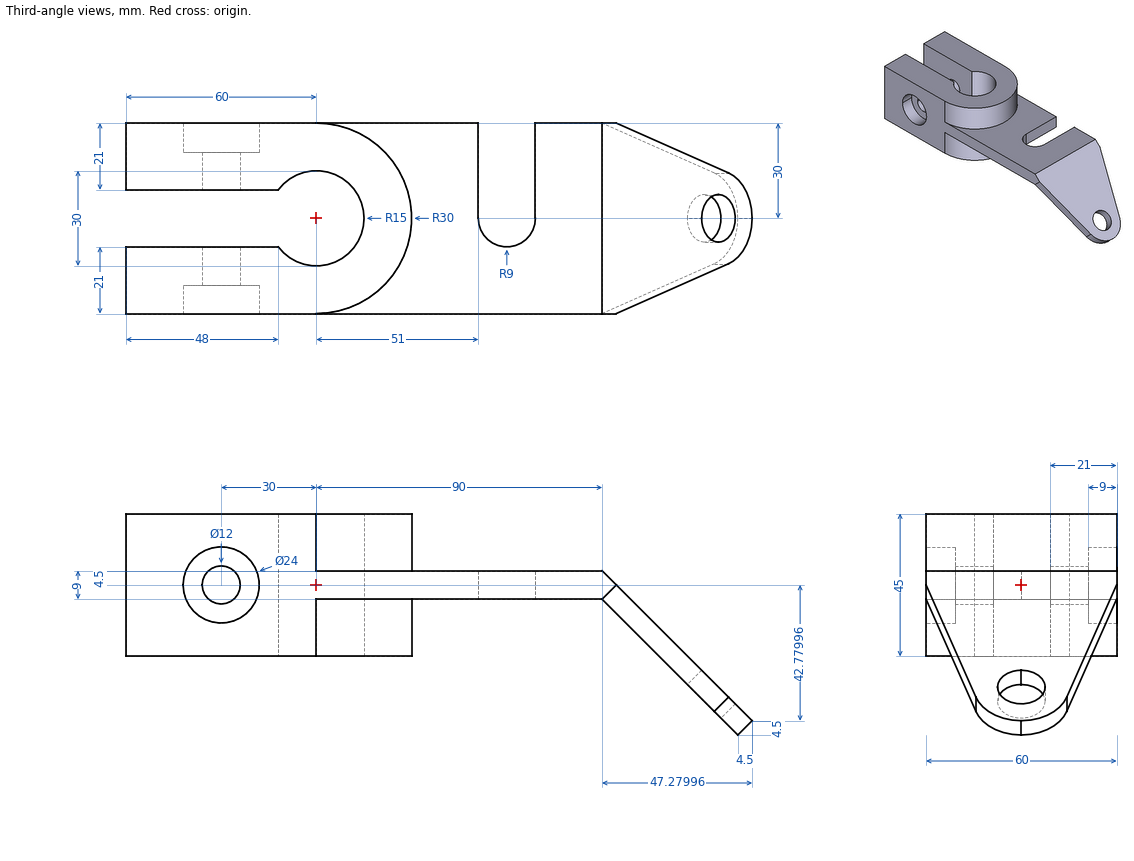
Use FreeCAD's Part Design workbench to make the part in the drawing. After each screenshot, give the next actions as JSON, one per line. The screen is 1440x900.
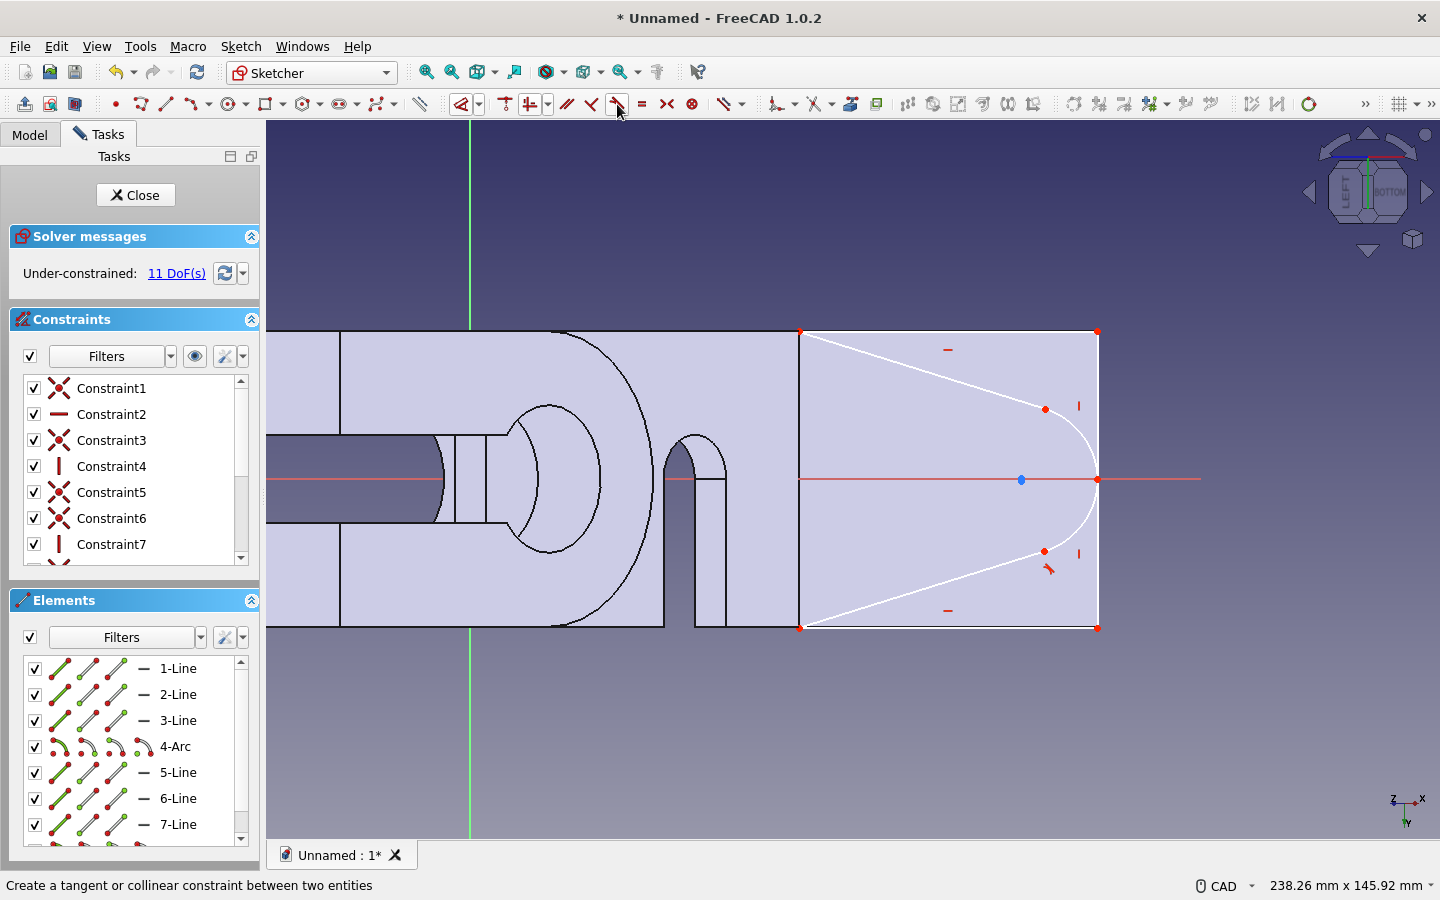
{"action": "left_click", "coordinate": [1098, 583]}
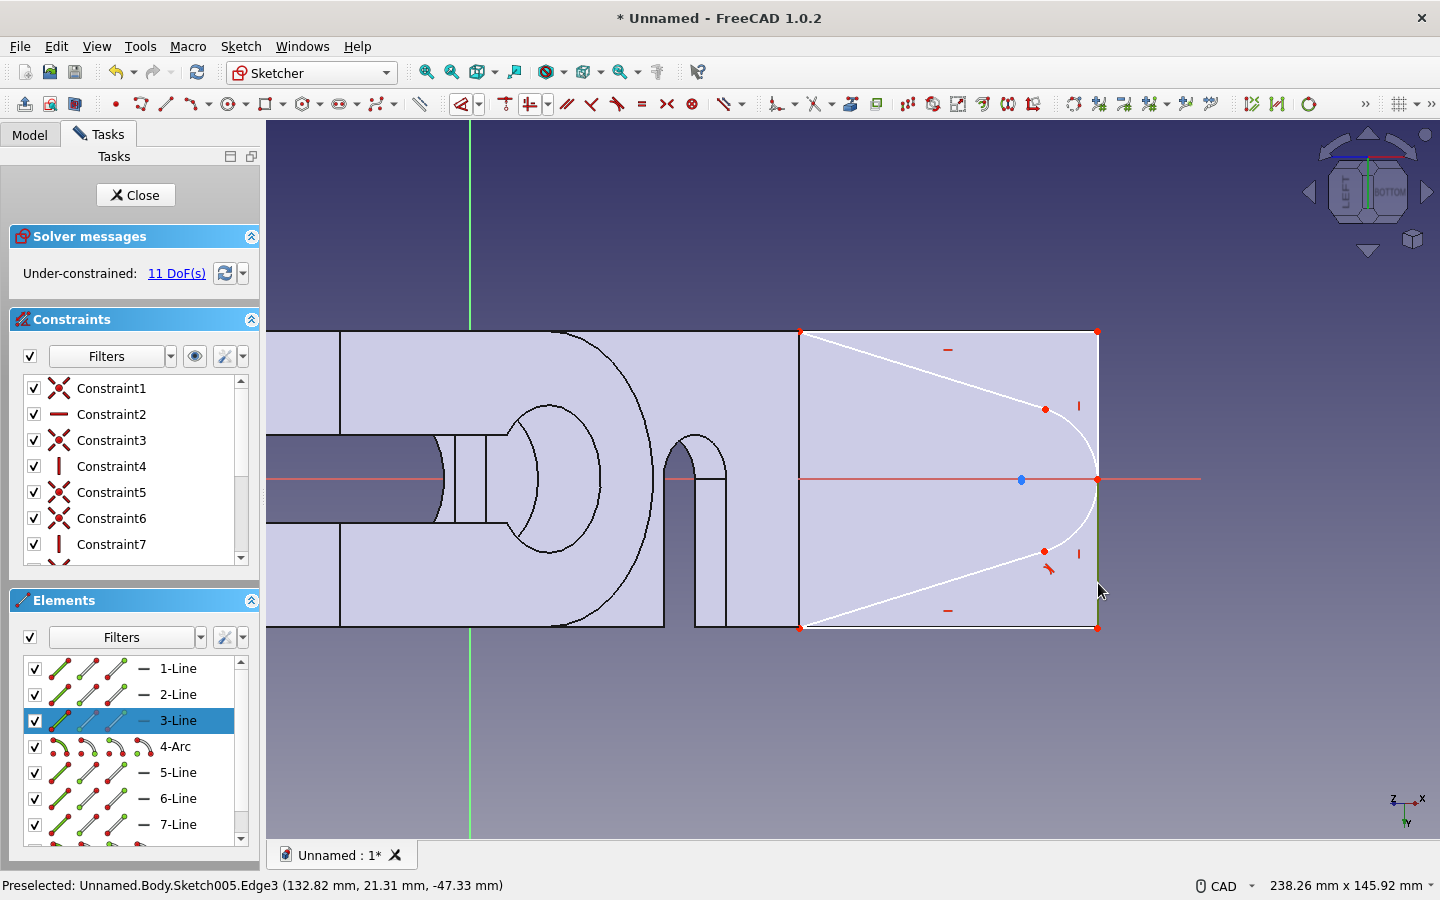
{"action": "left_click", "coordinate": [1070, 538]}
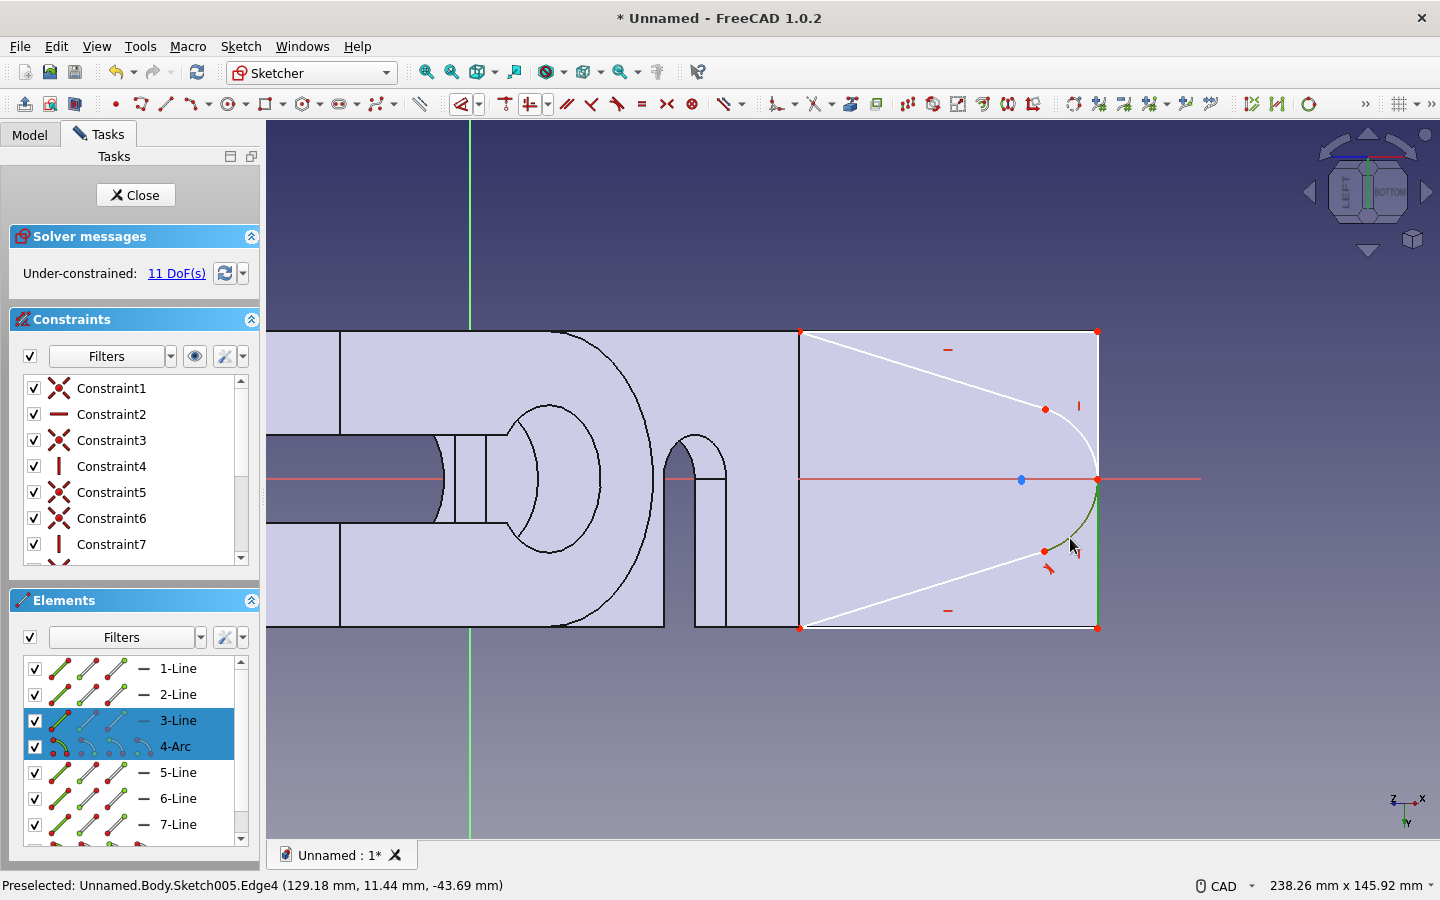
{"action": "left_click", "coordinate": [617, 104]}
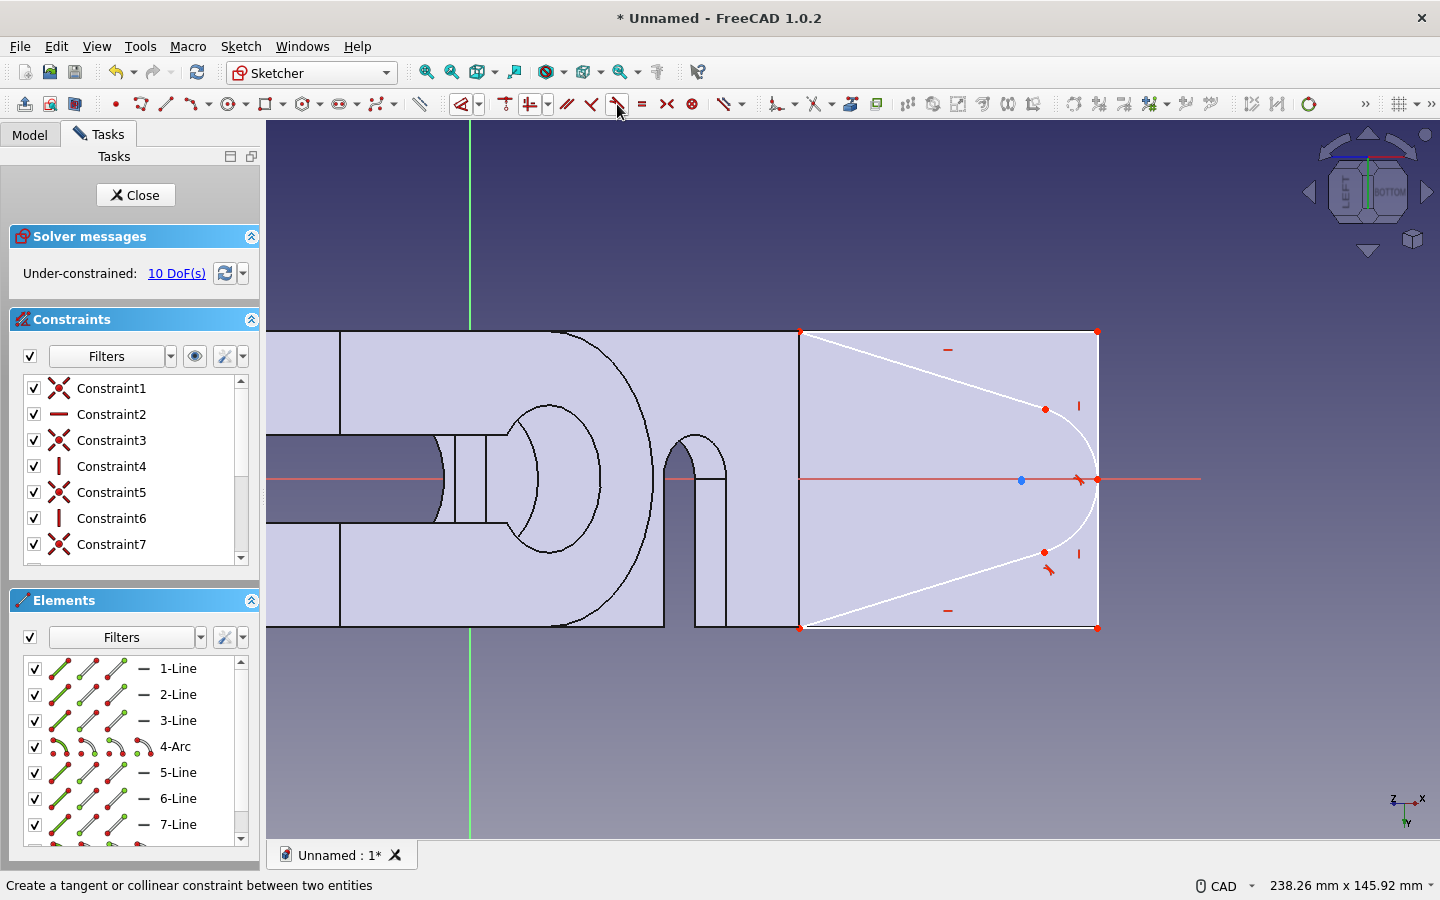
{"action": "left_click", "coordinate": [1098, 583]}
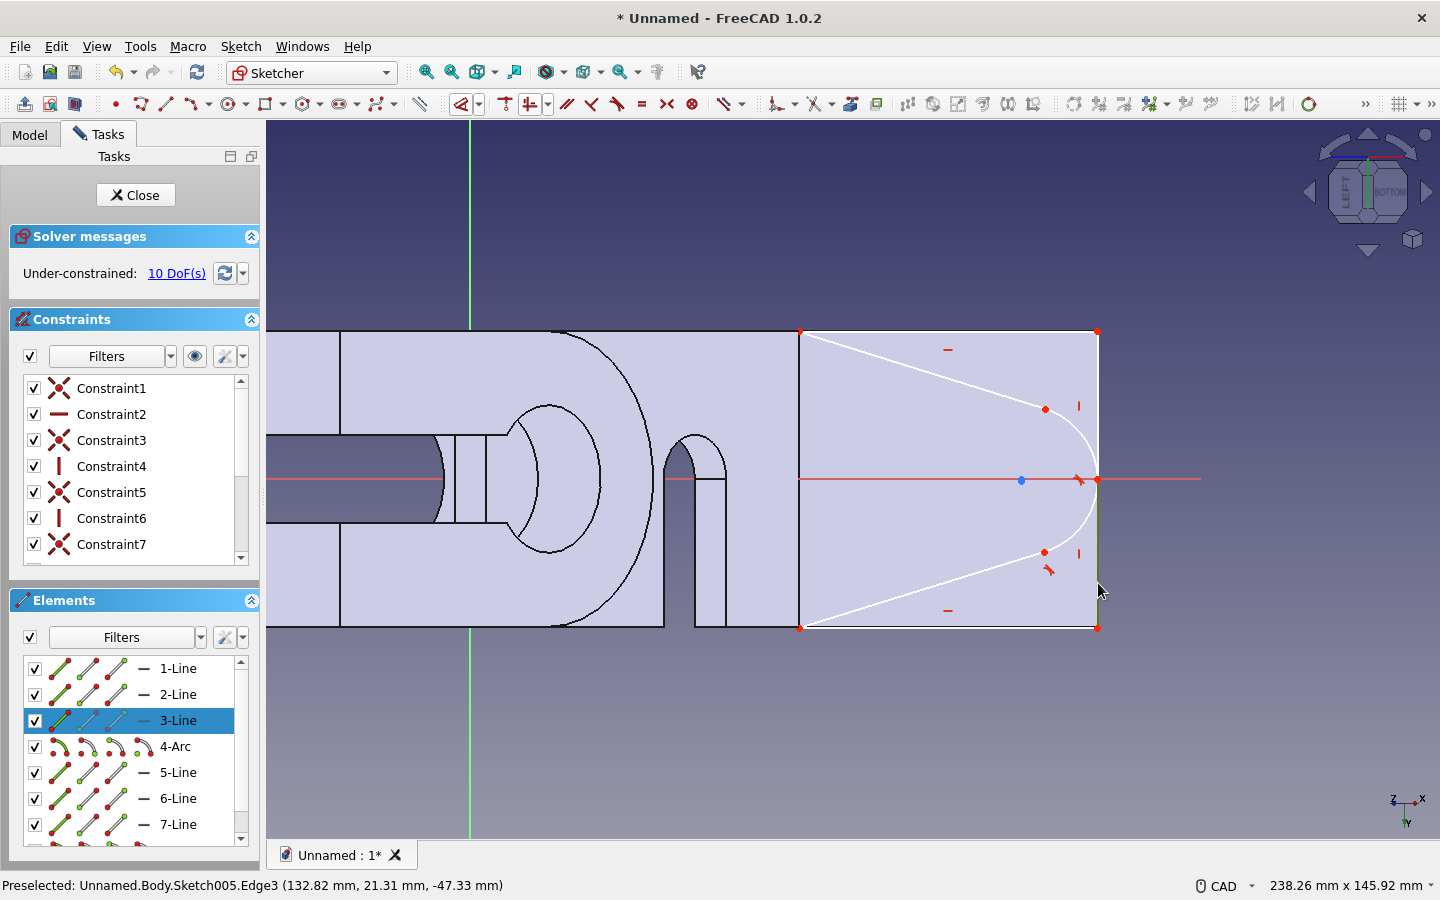
{"action": "left_click", "coordinate": [1070, 423]}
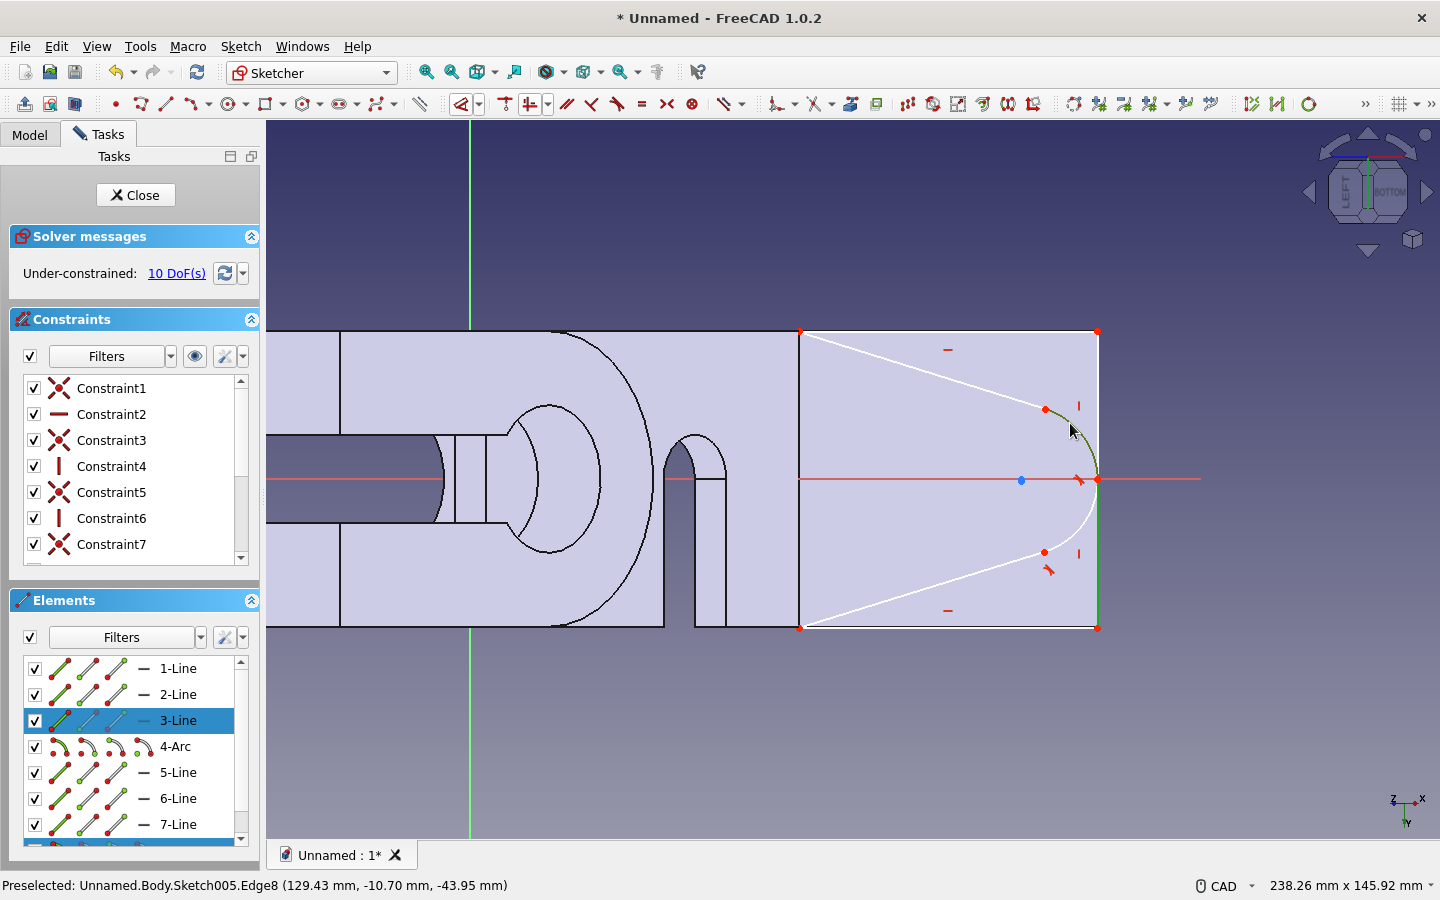
{"action": "left_click", "coordinate": [617, 104]}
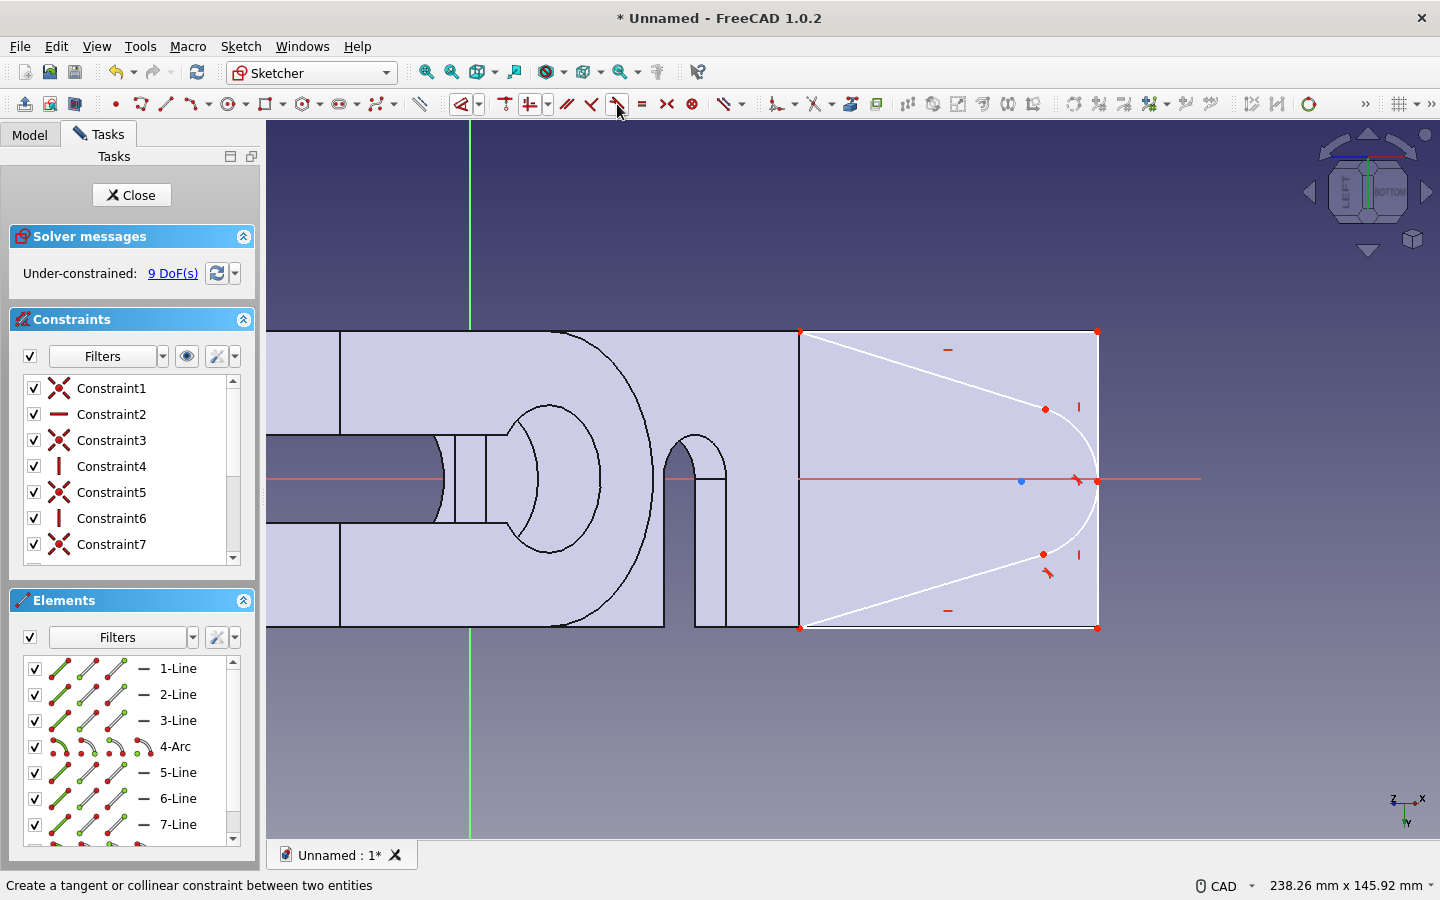
{"action": "left_click", "coordinate": [873, 355]}